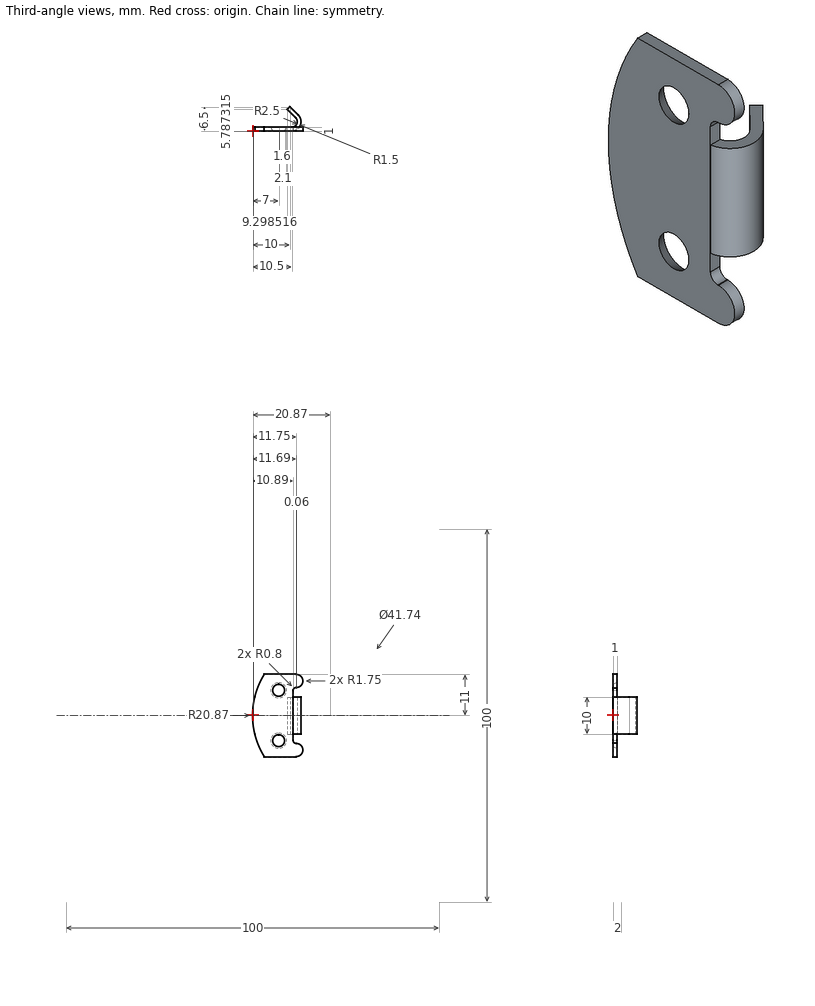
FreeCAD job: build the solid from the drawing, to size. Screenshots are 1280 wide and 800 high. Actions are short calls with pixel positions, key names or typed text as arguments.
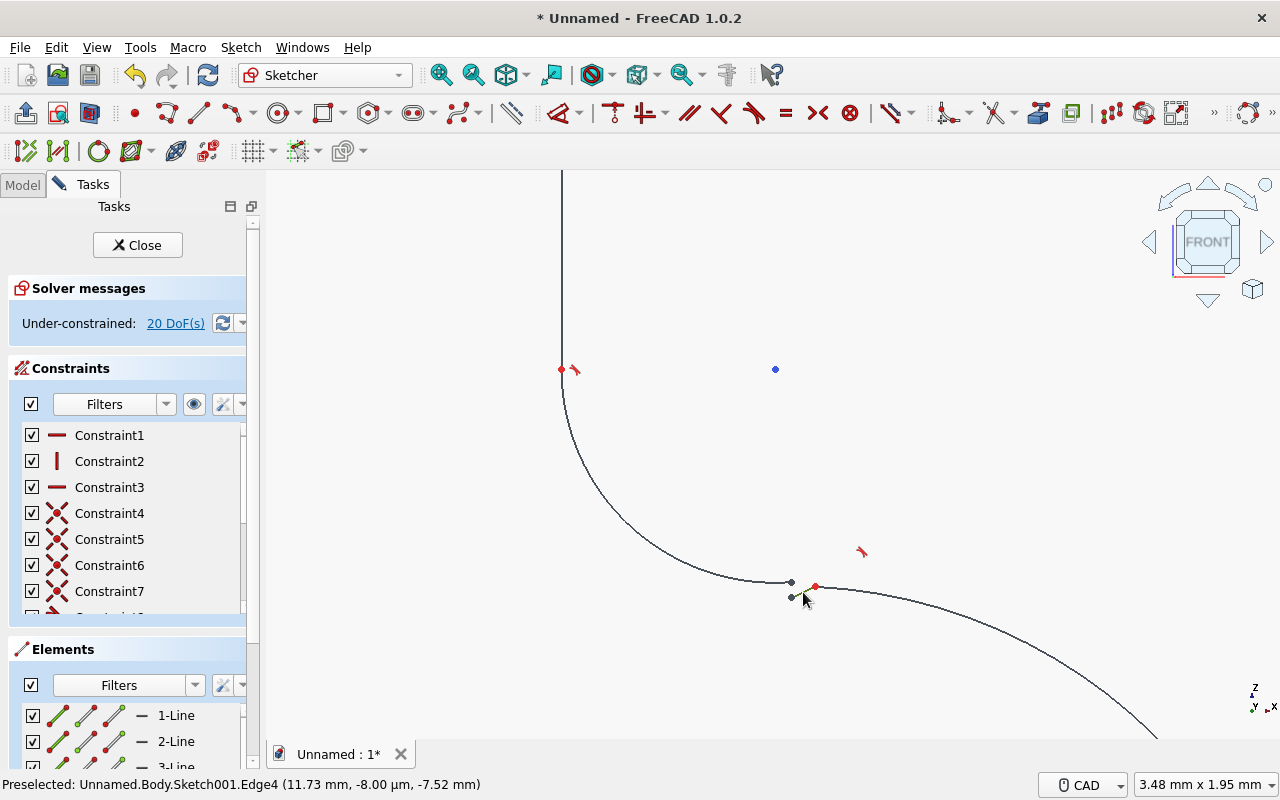
scroll(792, 587, down, 14)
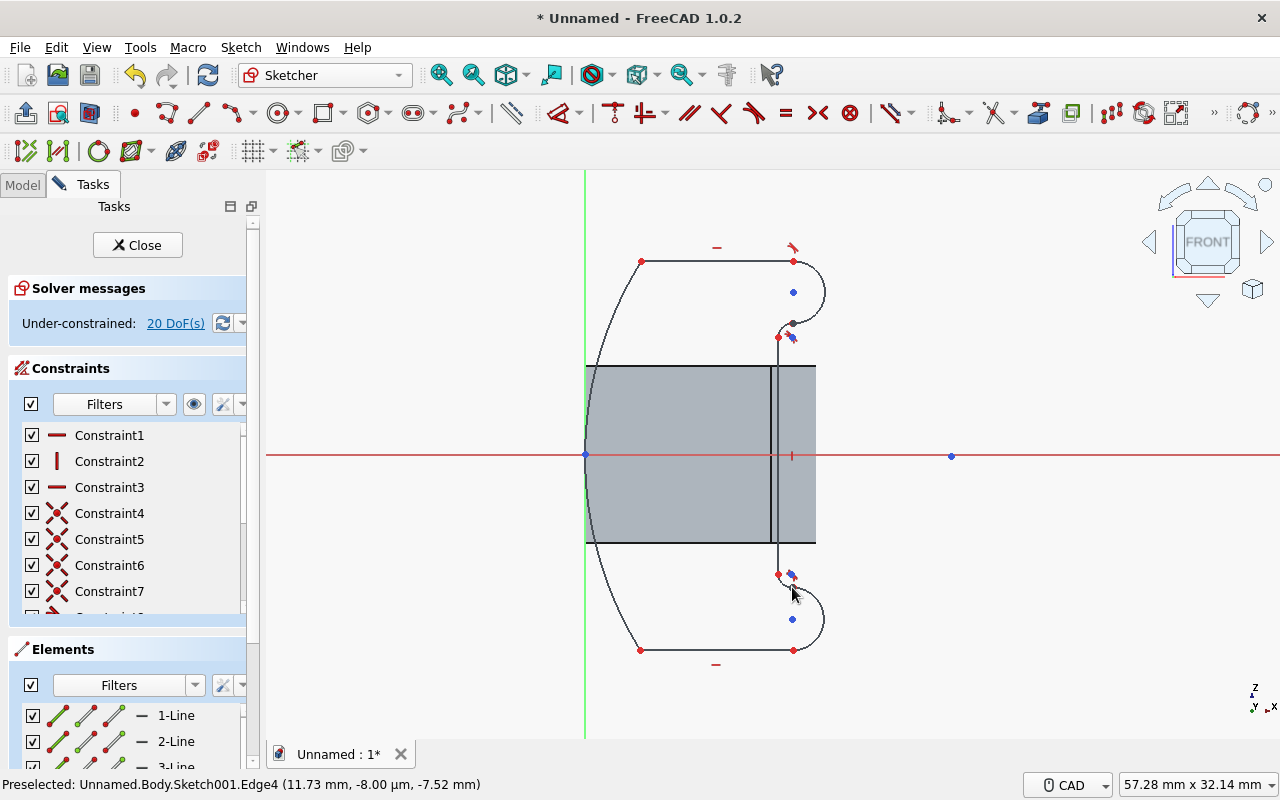
click(812, 594)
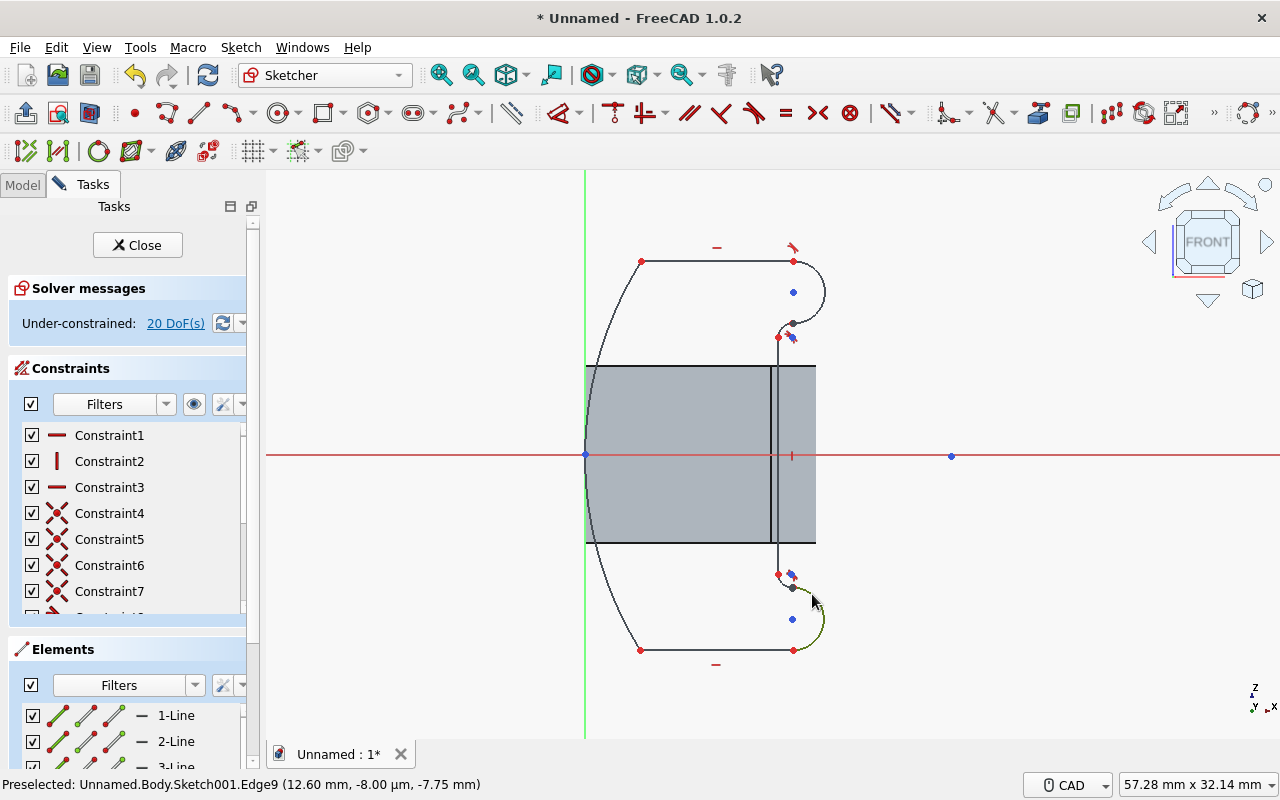
click(754, 114)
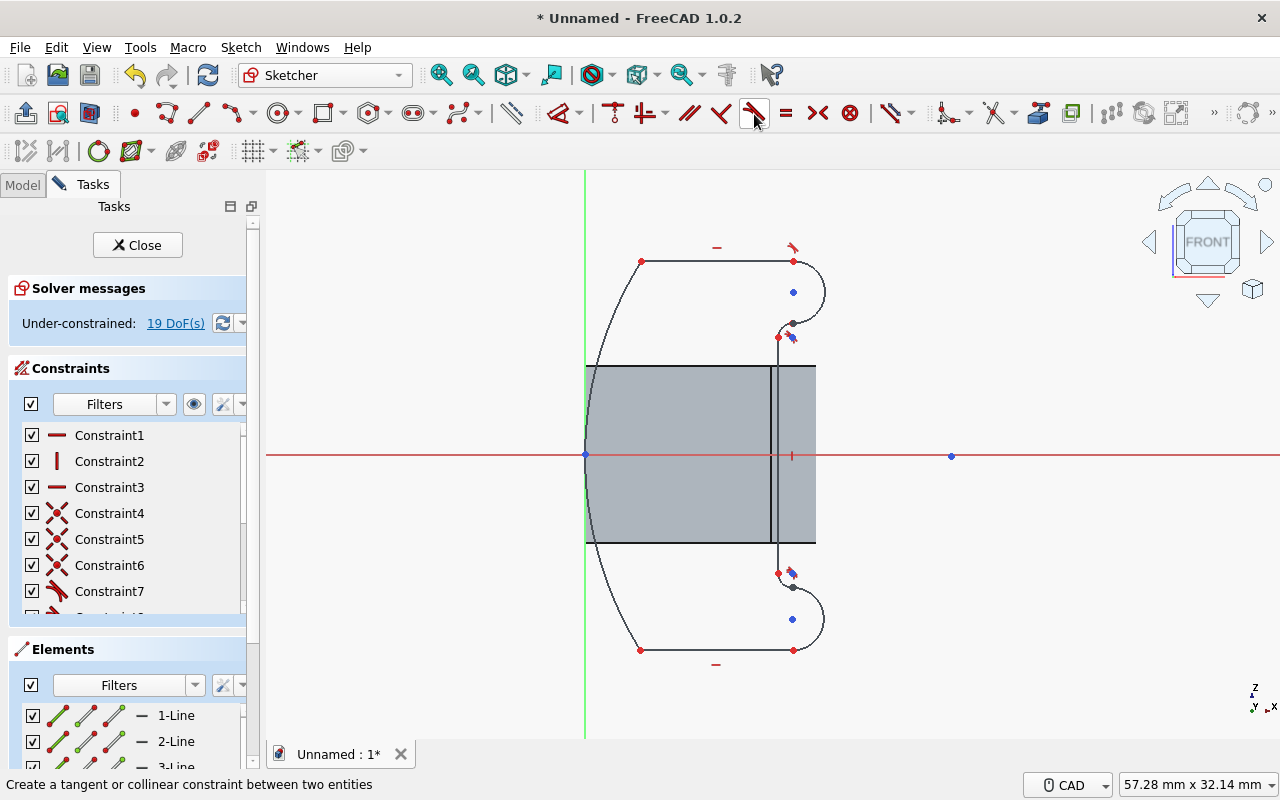
click(748, 650)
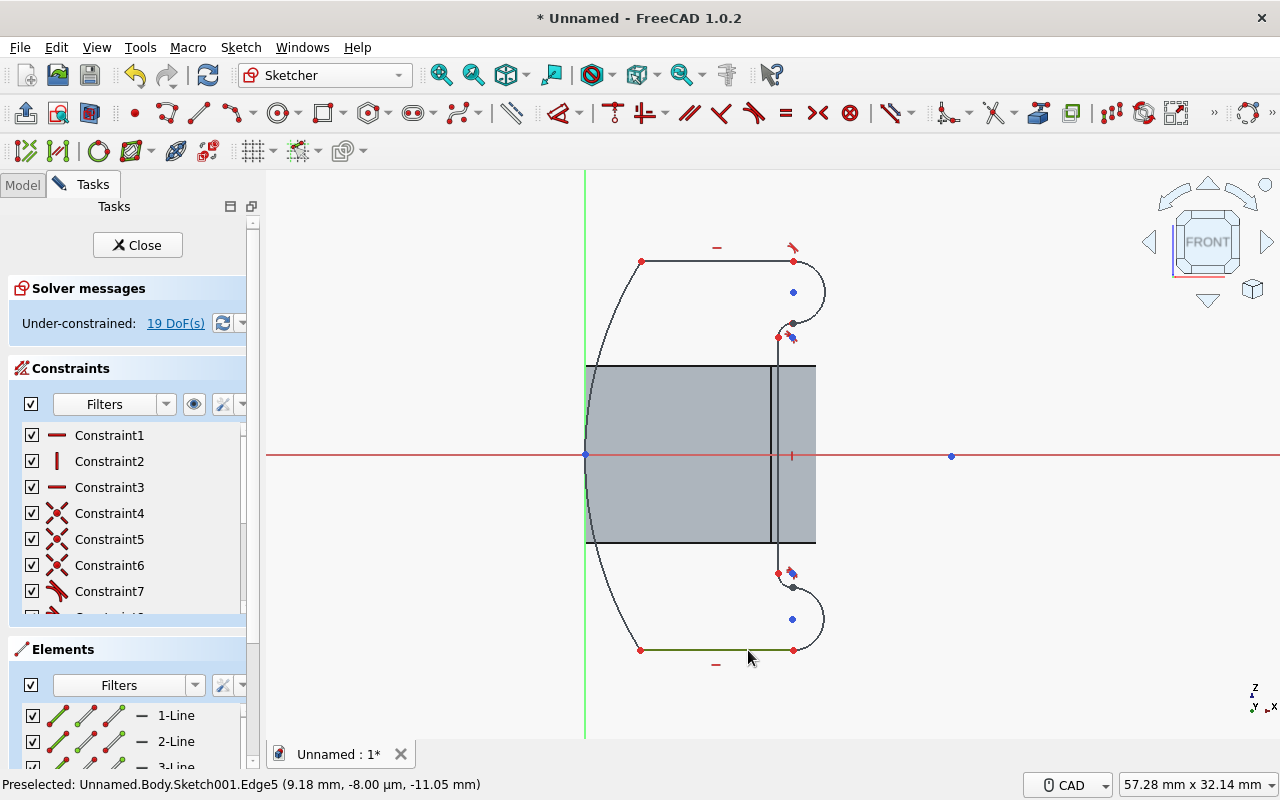
click(818, 637)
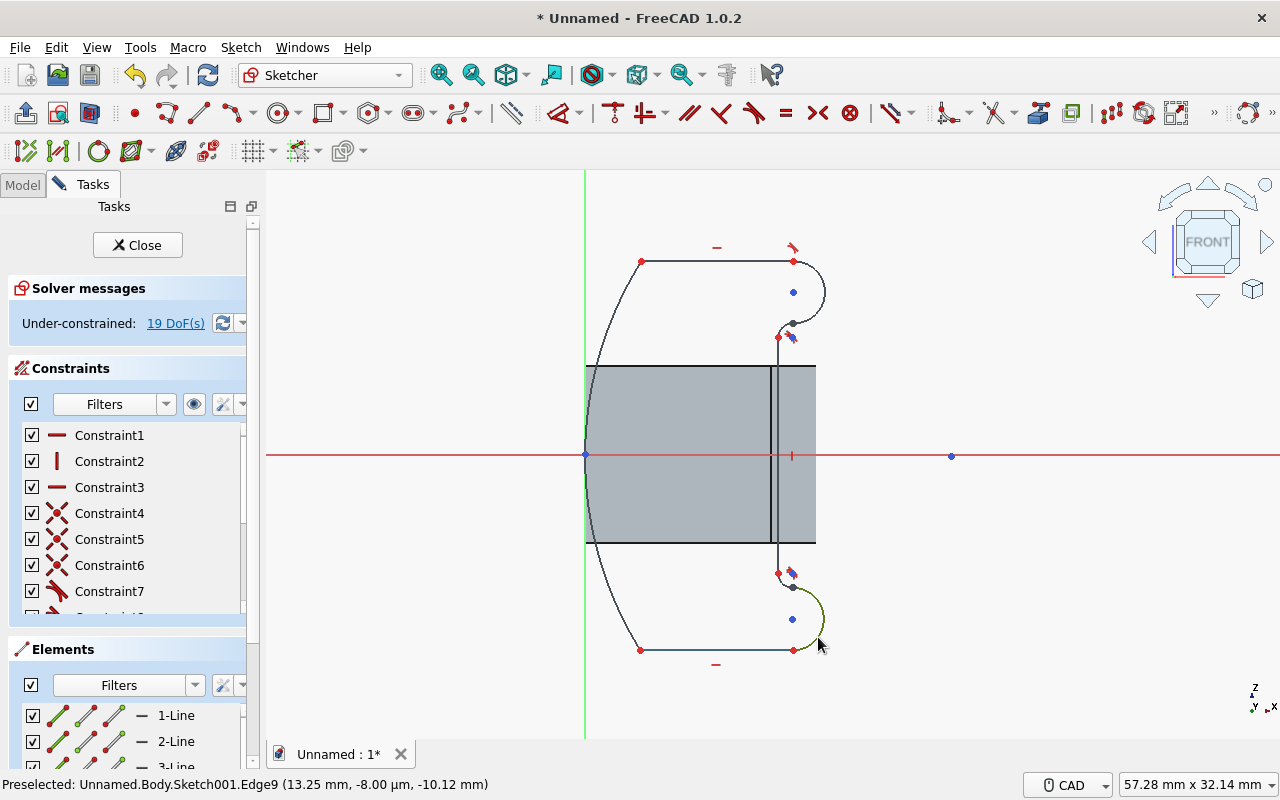
click(754, 114)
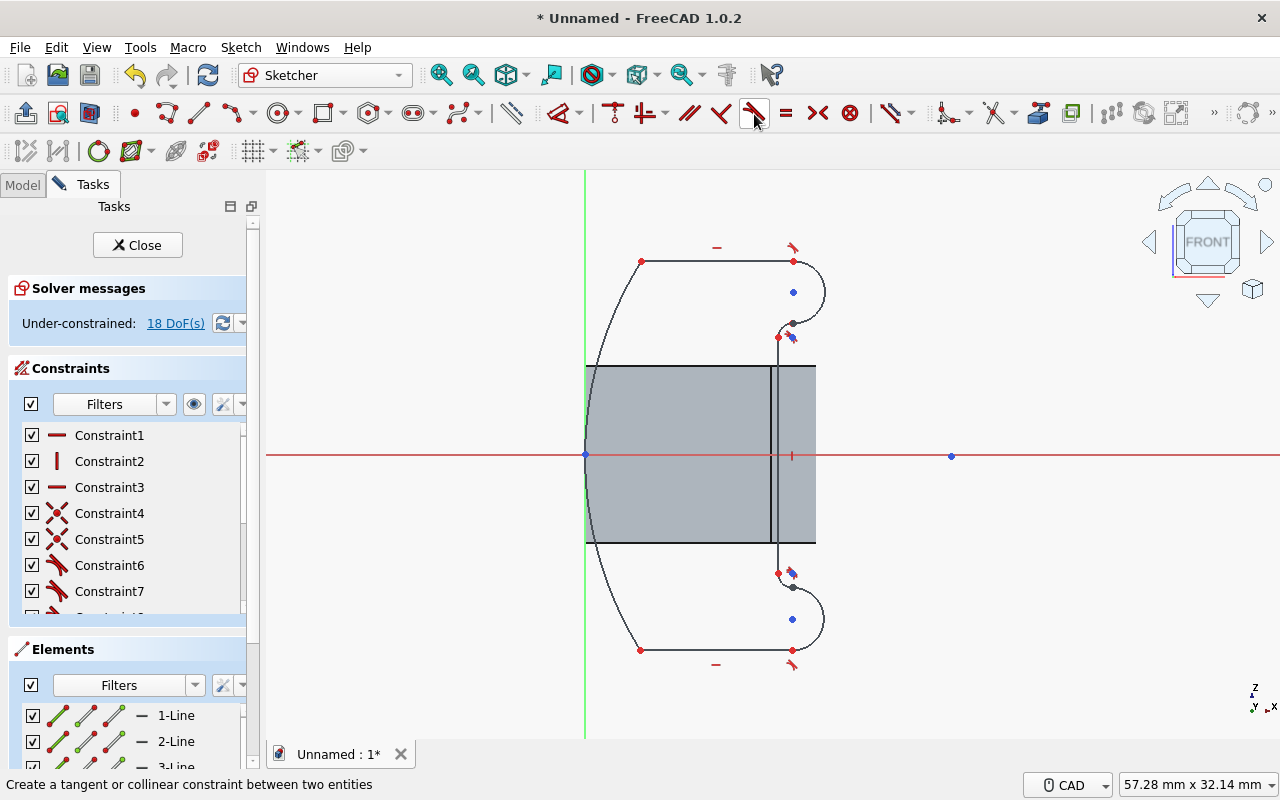
scroll(783, 327, up, 2)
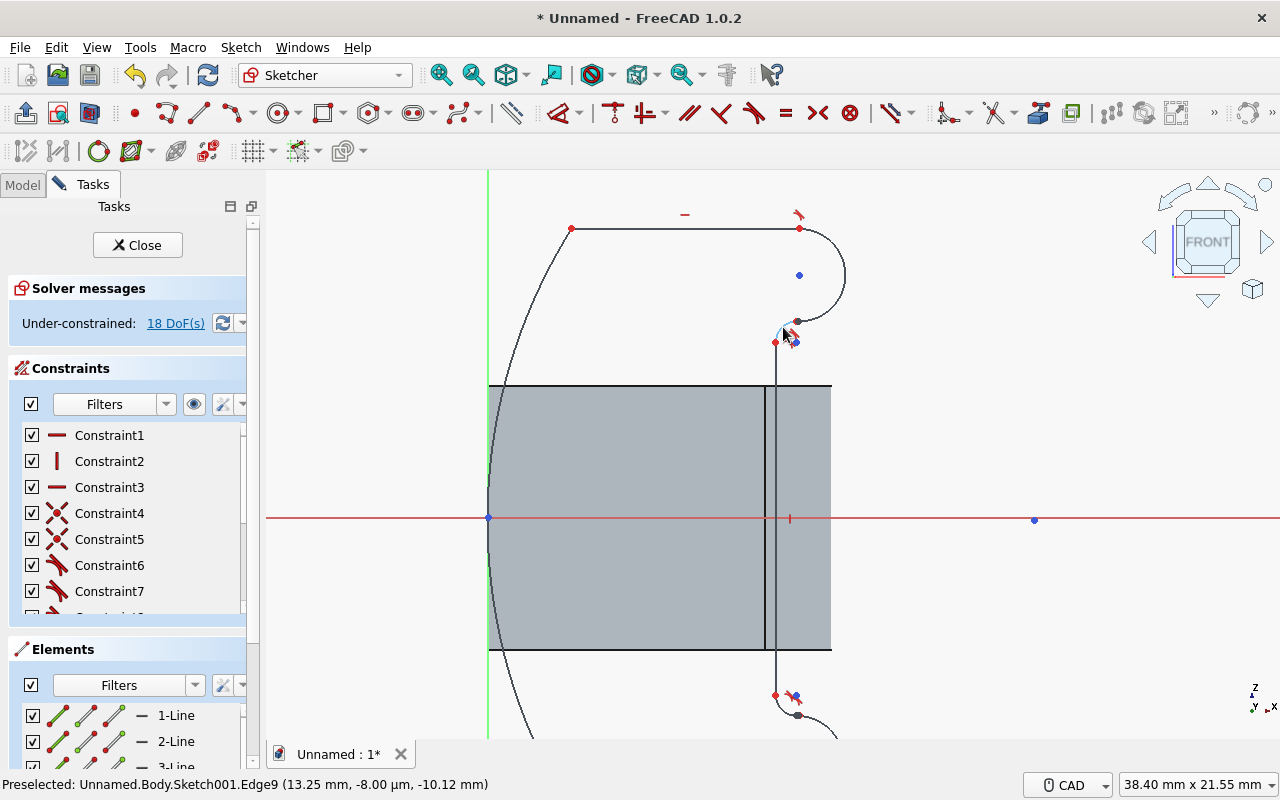
click(782, 327)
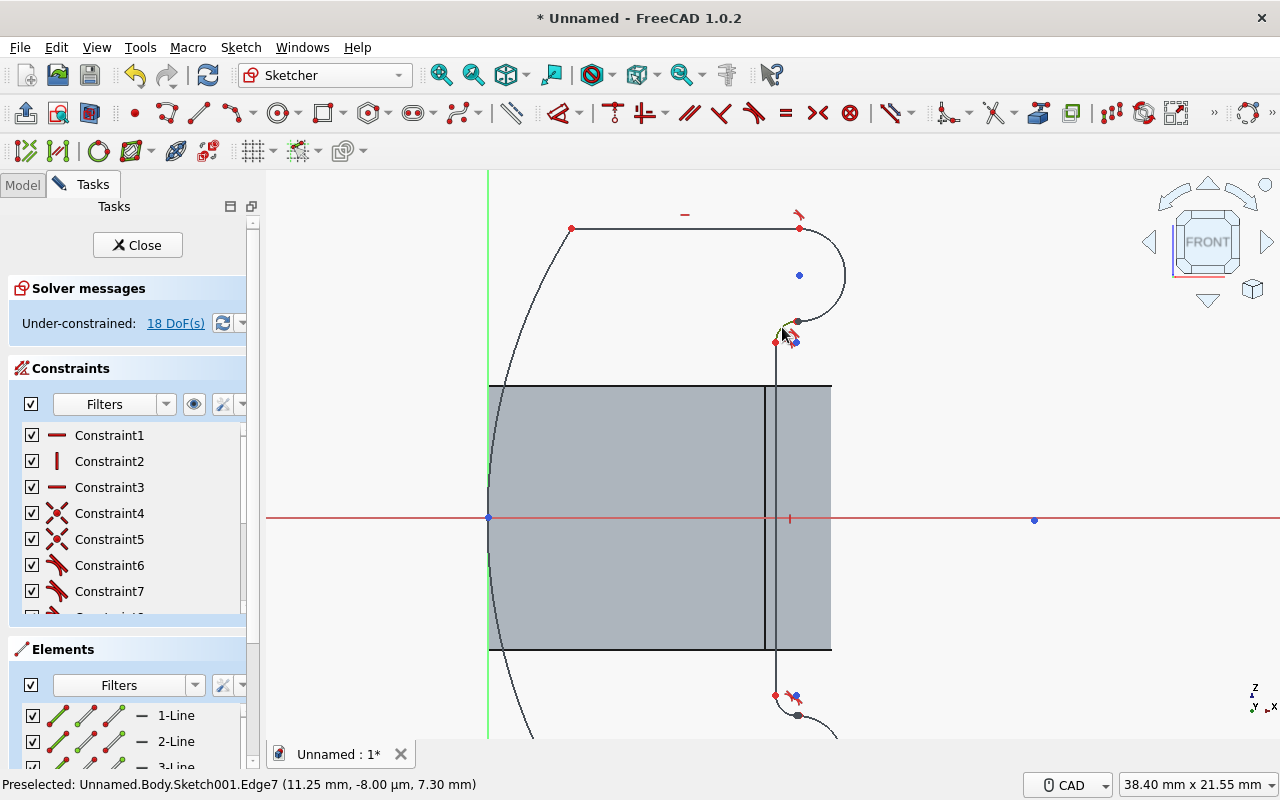
scroll(778, 705, up, 2)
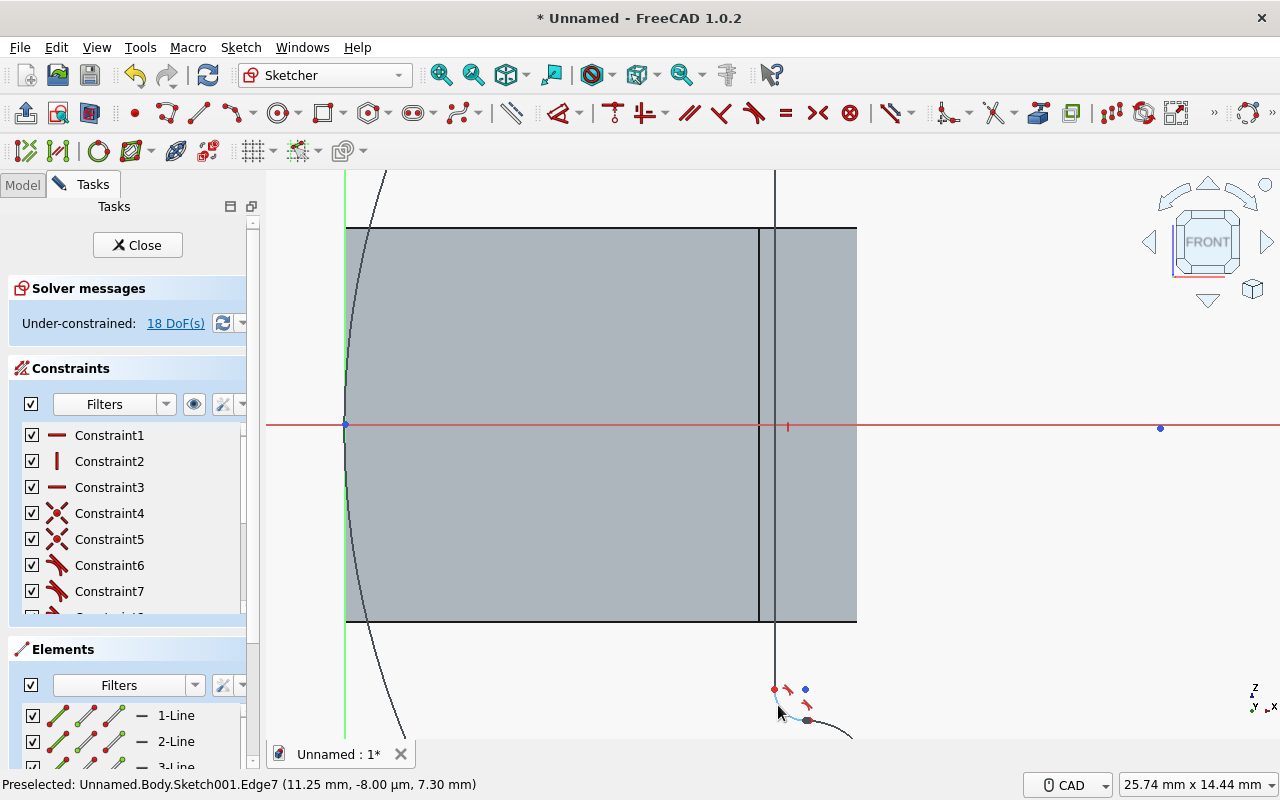
click(778, 705)